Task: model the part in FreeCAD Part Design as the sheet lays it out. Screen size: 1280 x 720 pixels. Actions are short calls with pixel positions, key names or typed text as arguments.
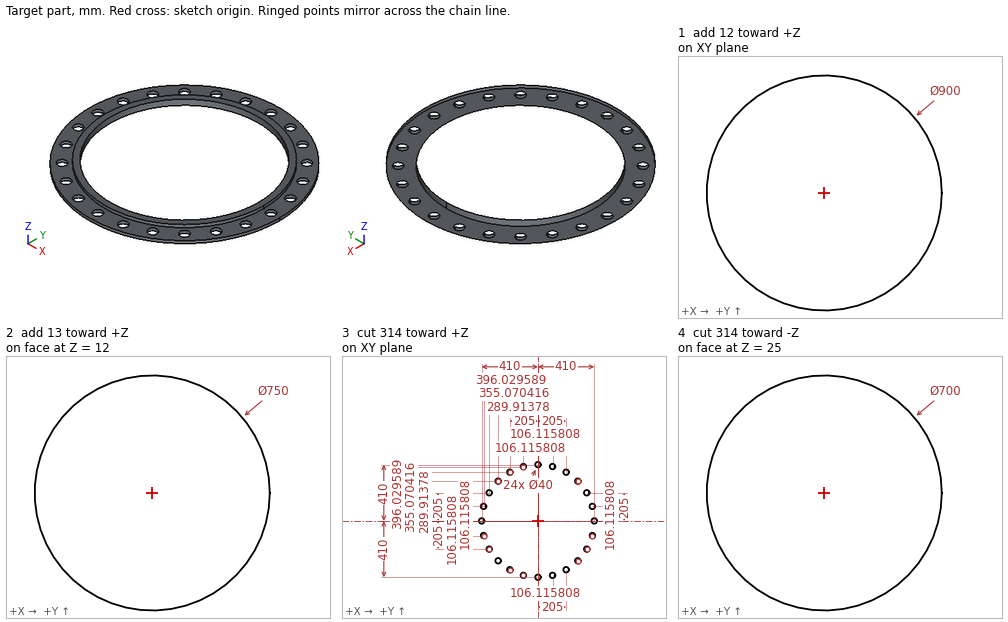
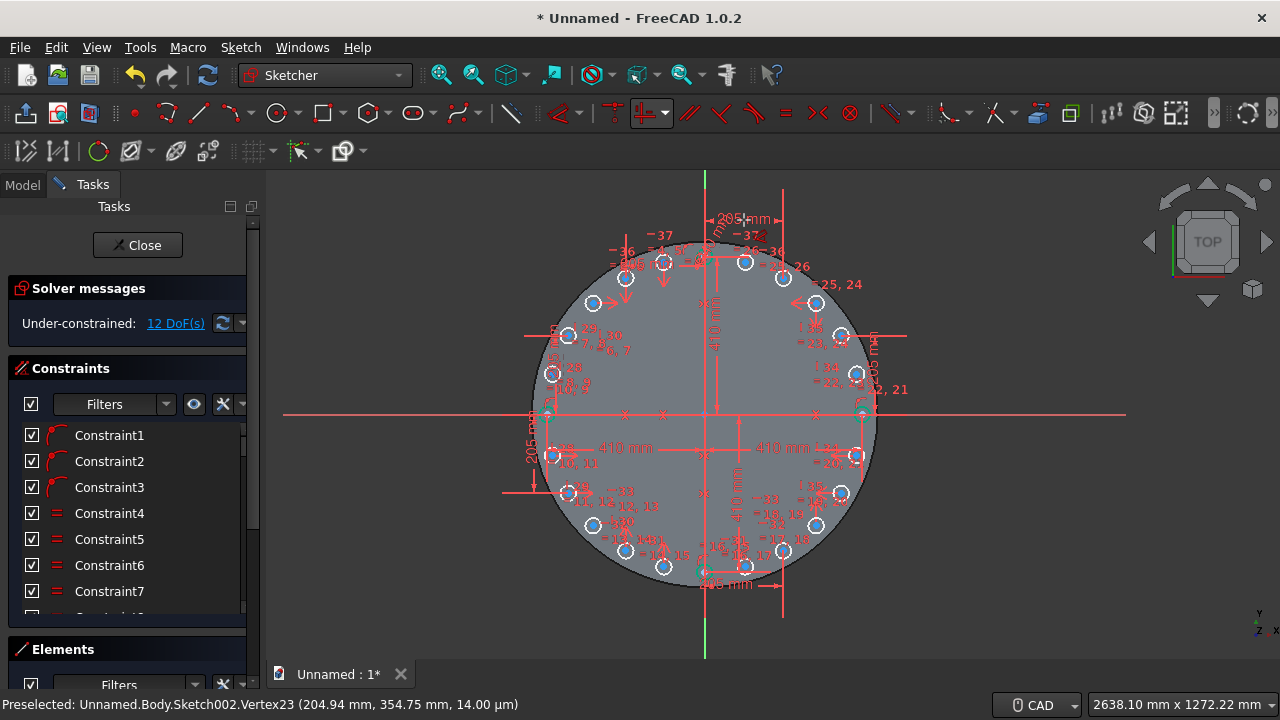
click(593, 303)
click(623, 245)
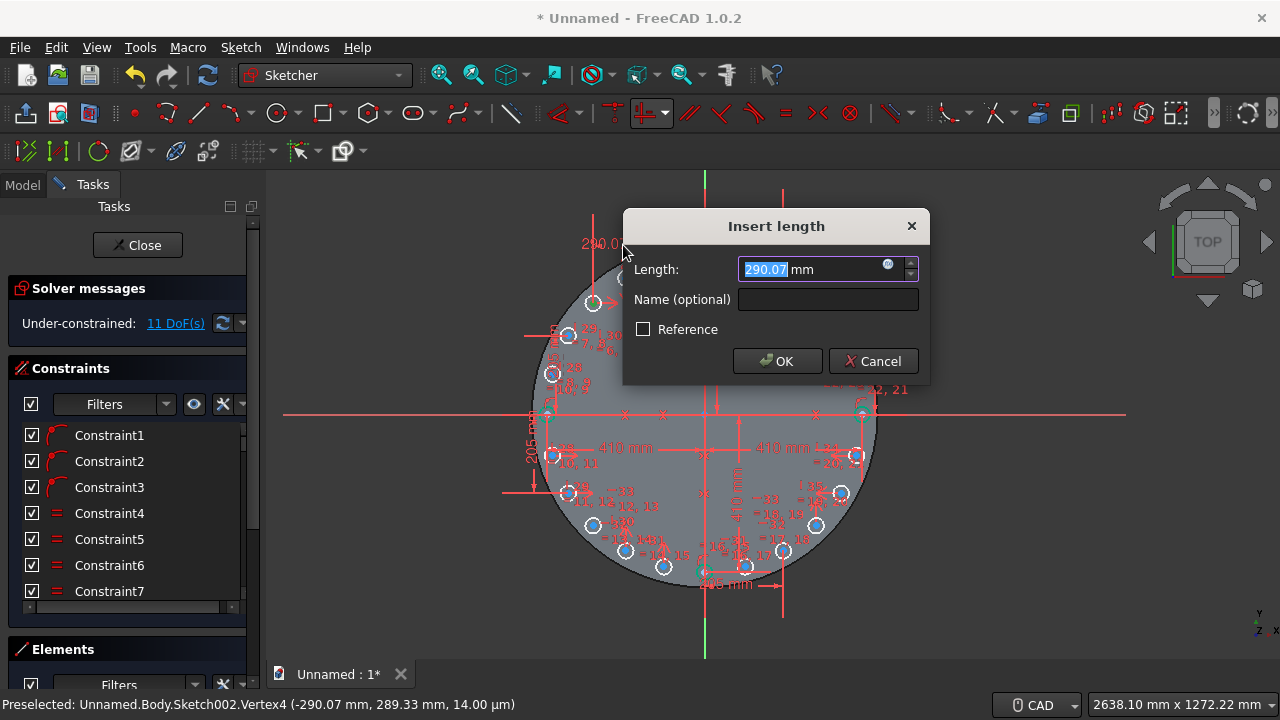
text(289.91378)
key(Return)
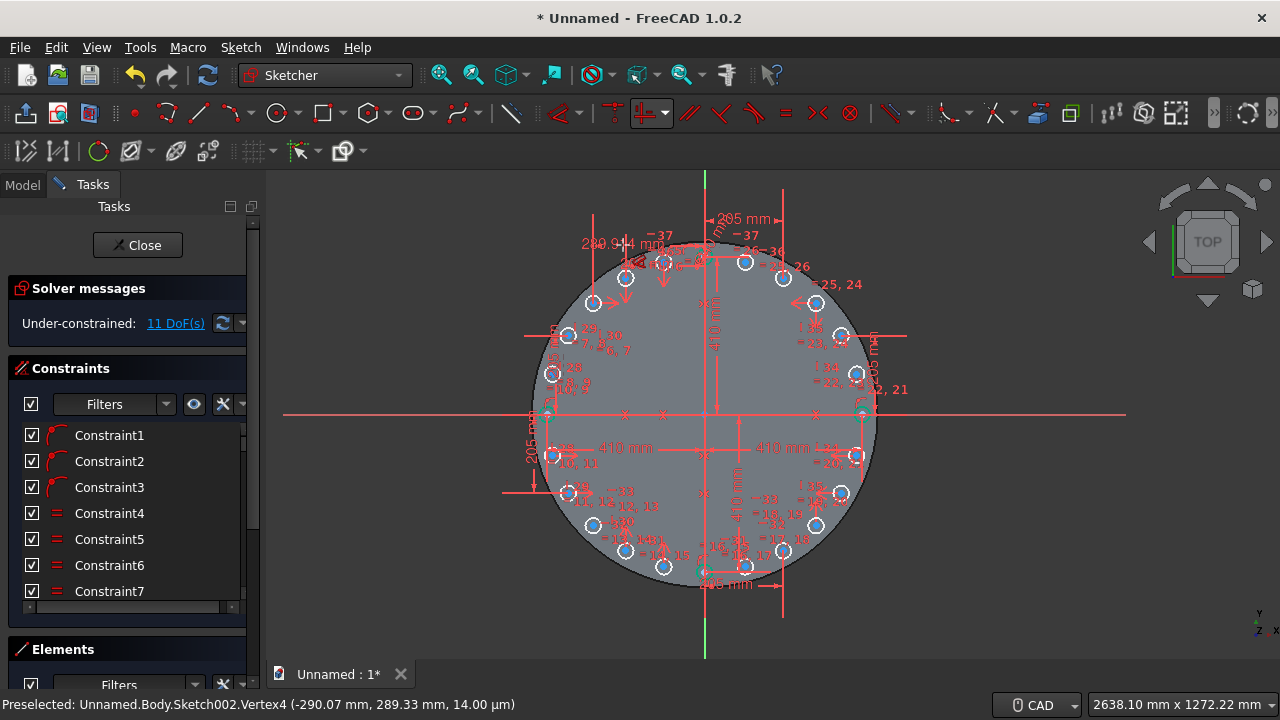
click(593, 303)
click(739, 359)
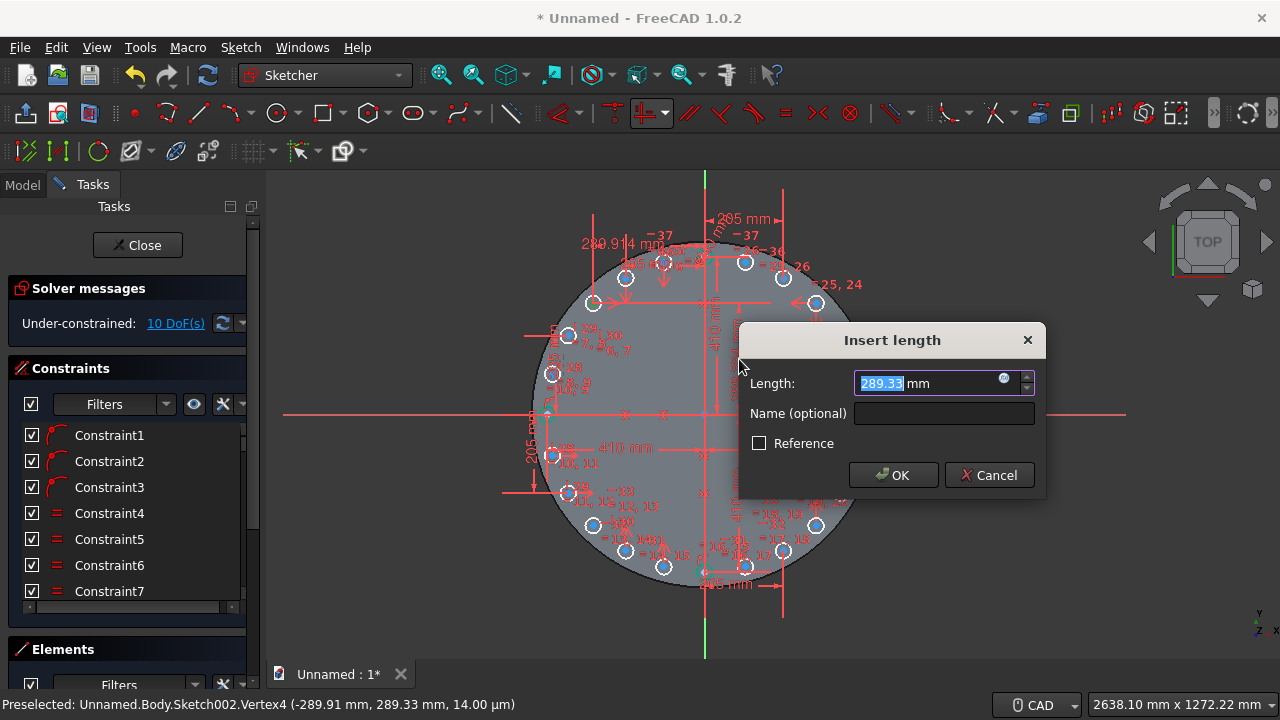
text(289.91378)
key(Return)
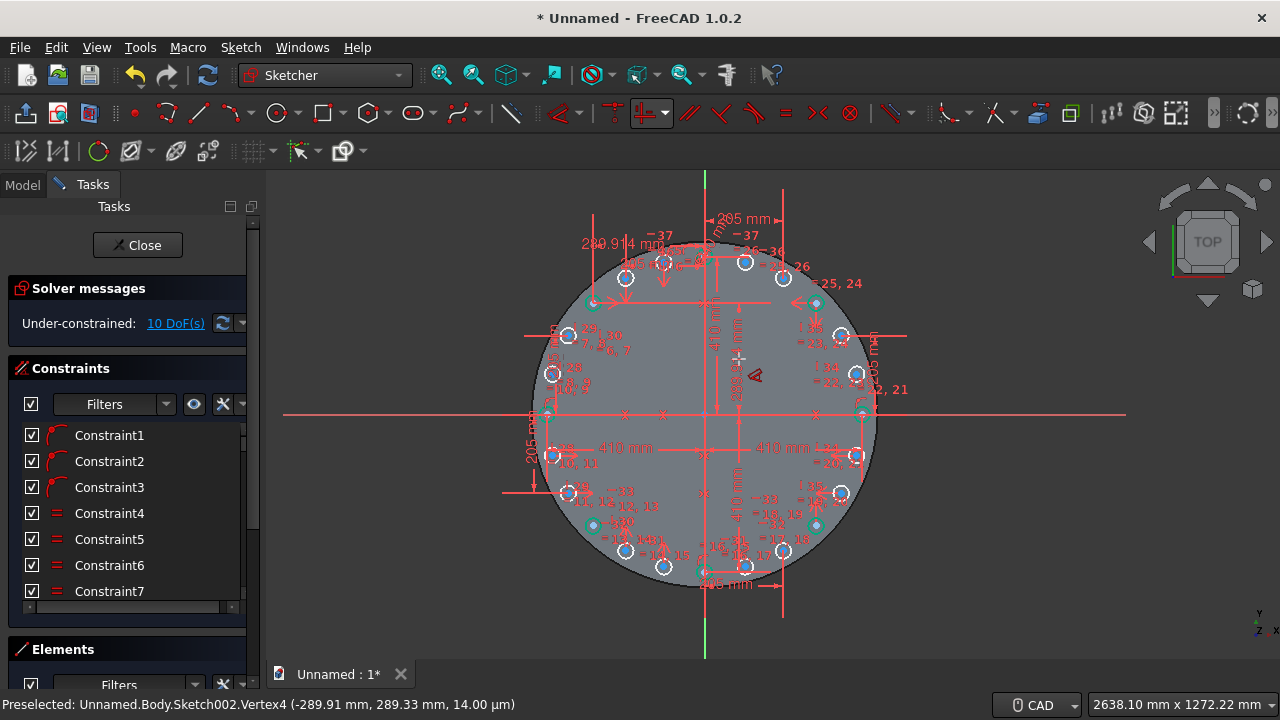
click(664, 262)
click(670, 204)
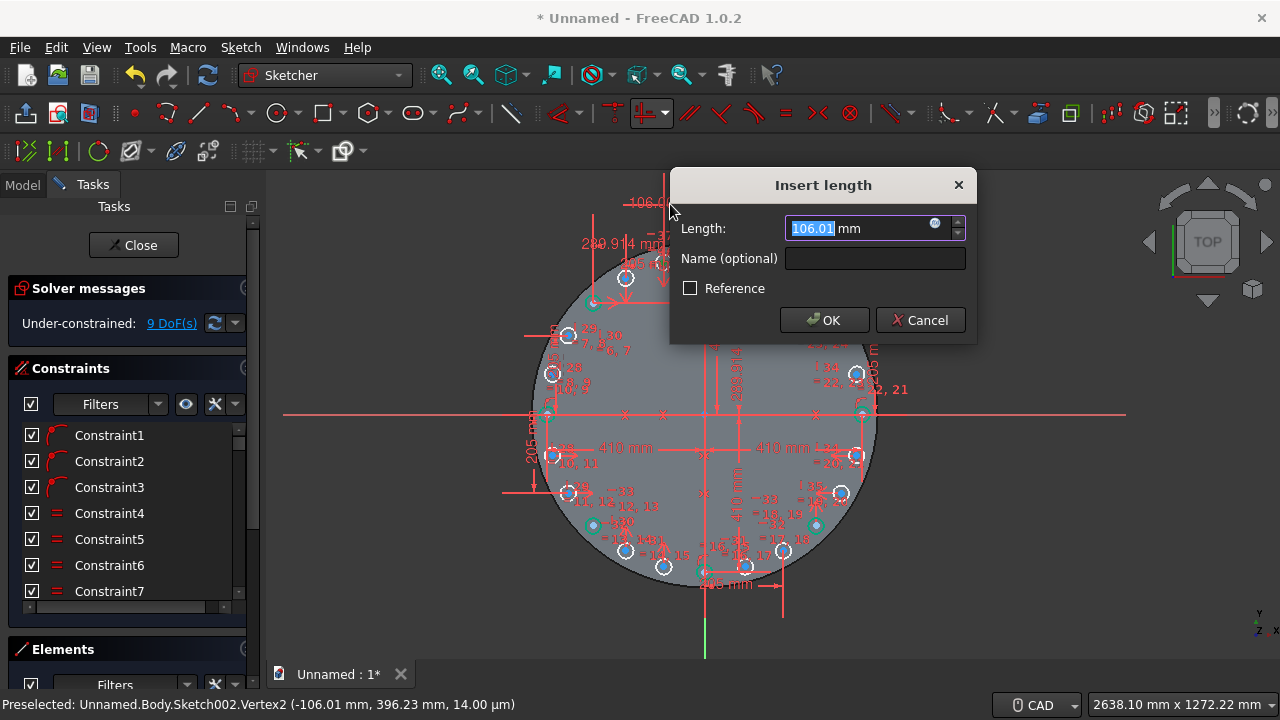
text(106.115808)
key(Return)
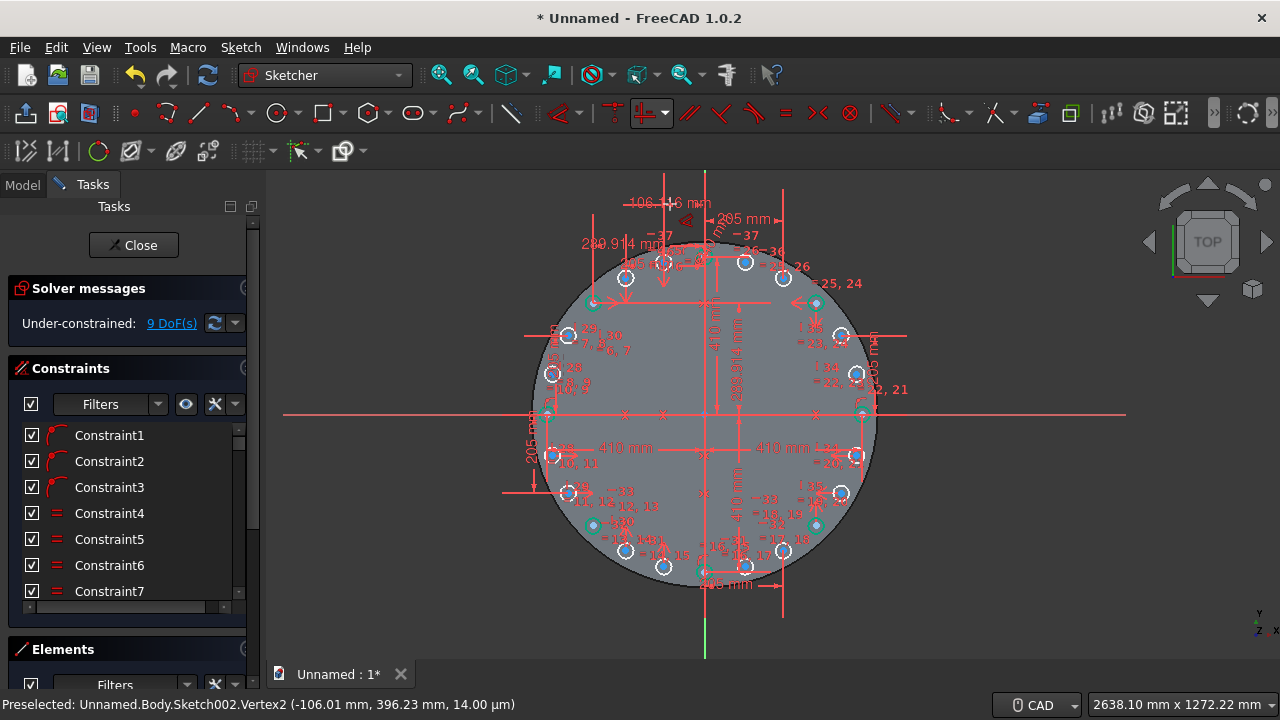
click(664, 262)
click(630, 338)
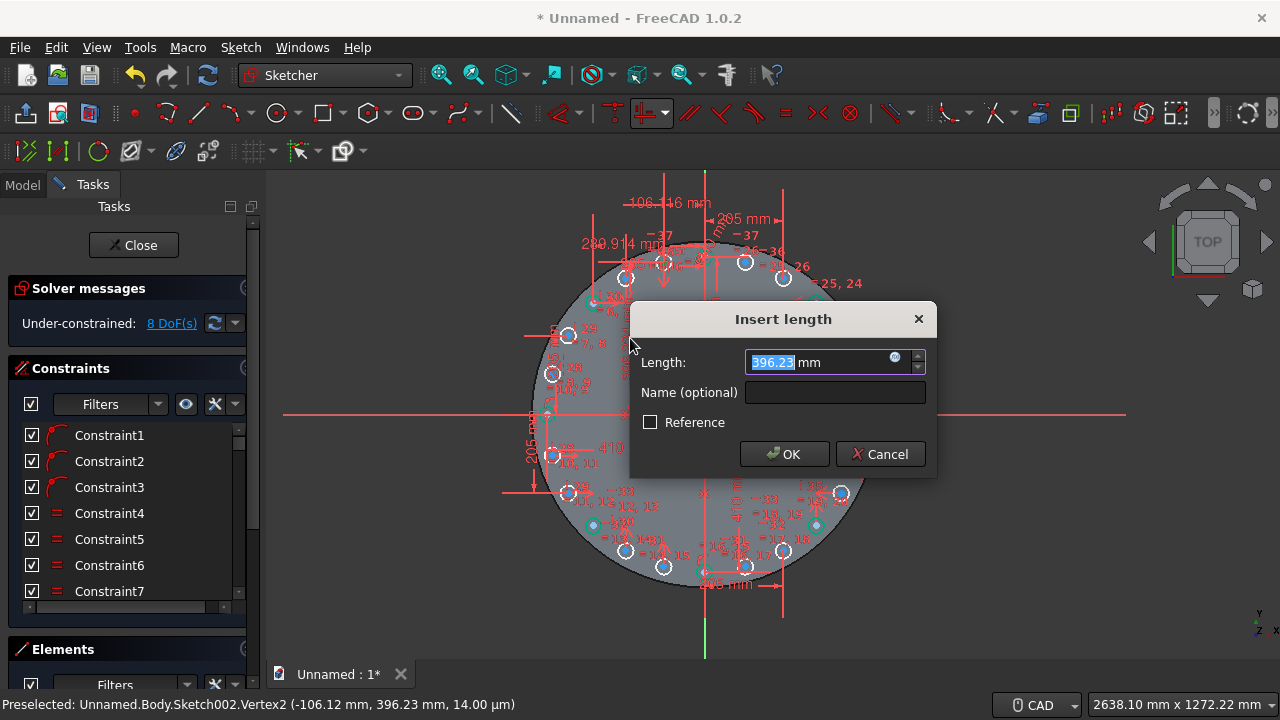
text(396.029589)
key(Return)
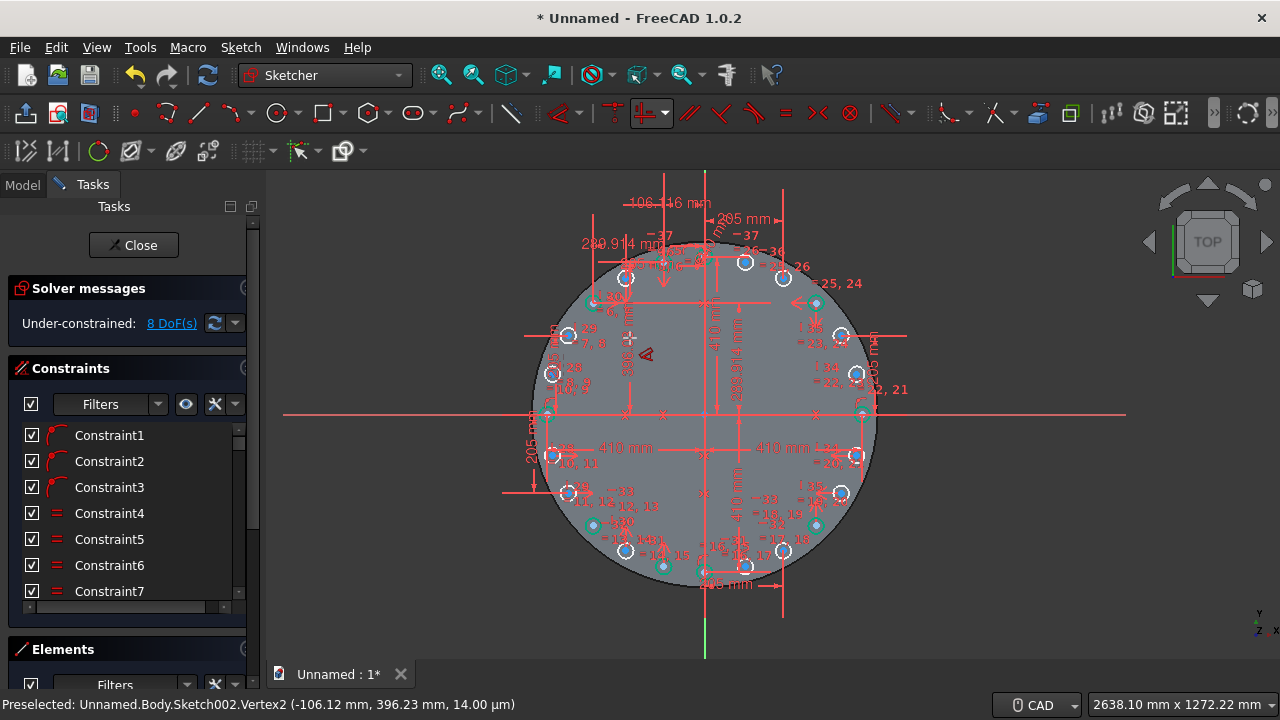
click(626, 278)
click(592, 378)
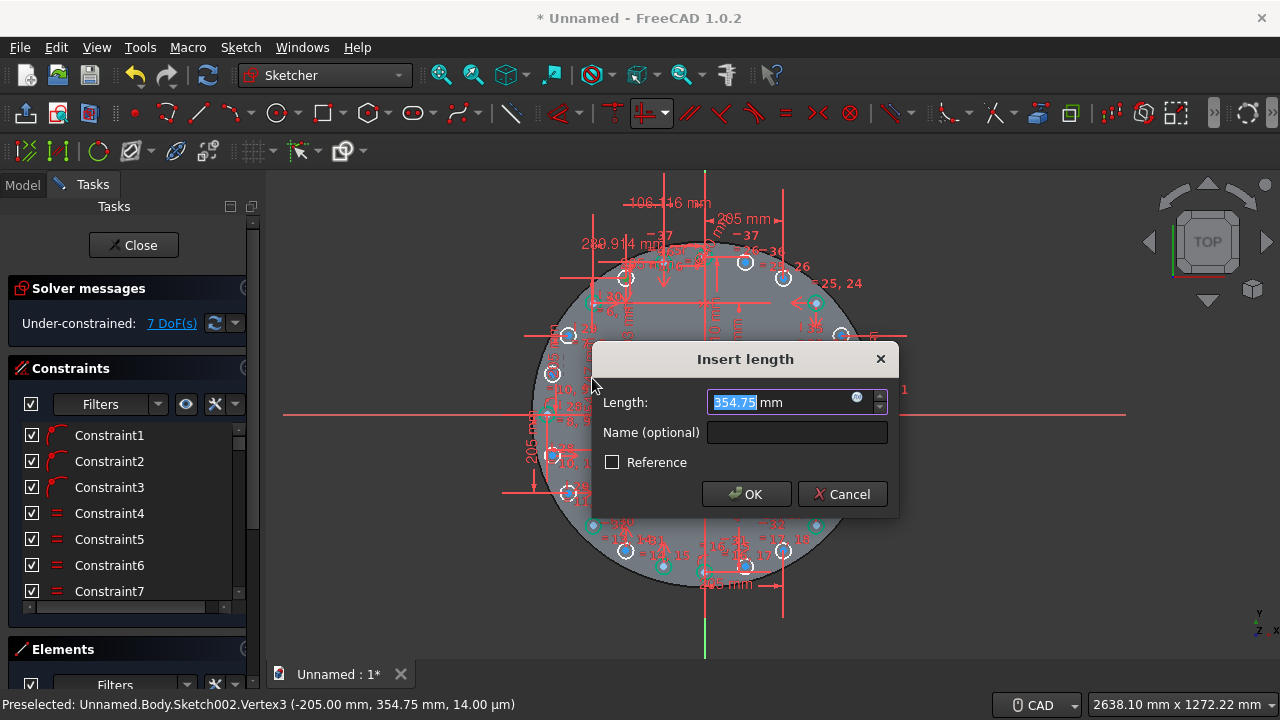
text(355.070416)
key(Return)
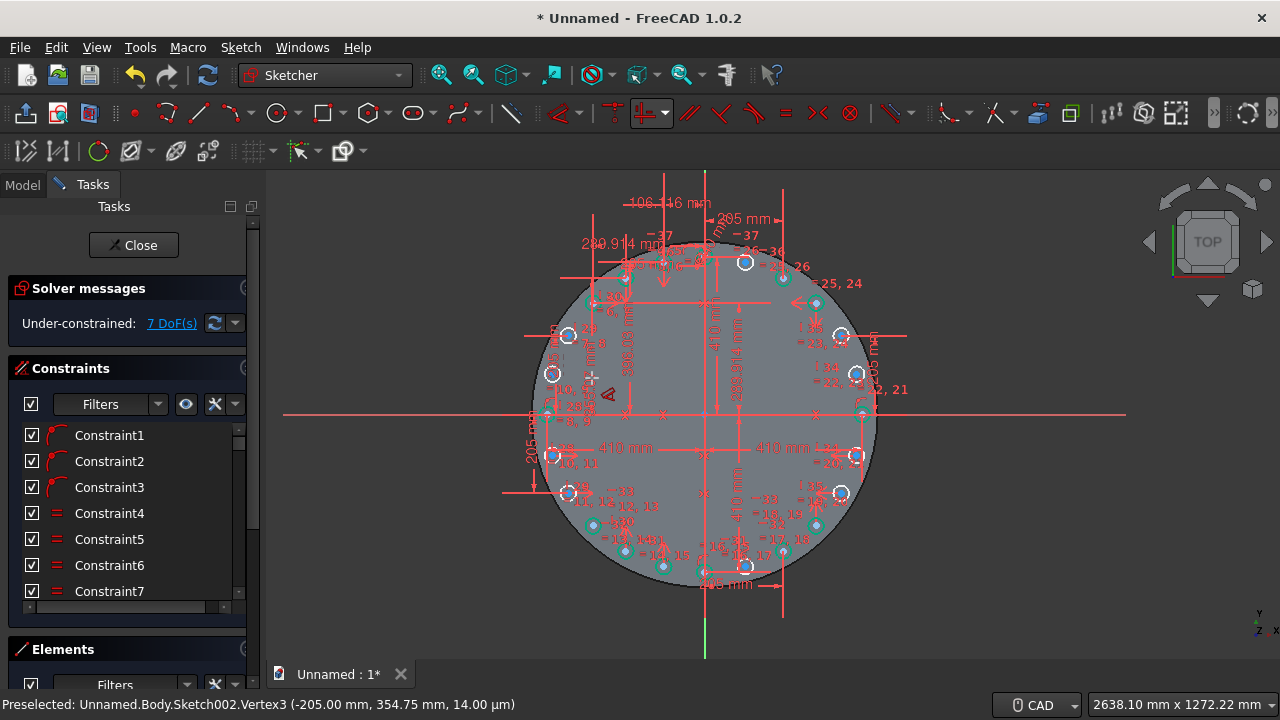
click(568, 336)
click(636, 302)